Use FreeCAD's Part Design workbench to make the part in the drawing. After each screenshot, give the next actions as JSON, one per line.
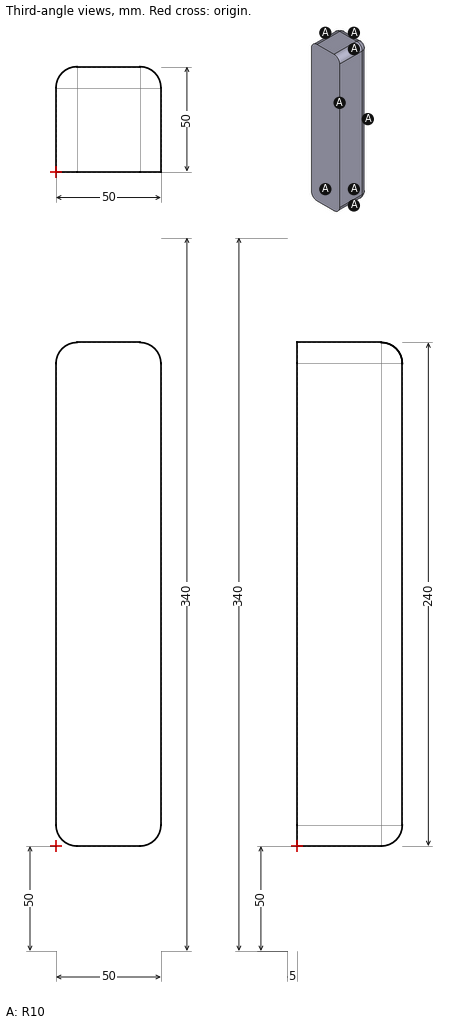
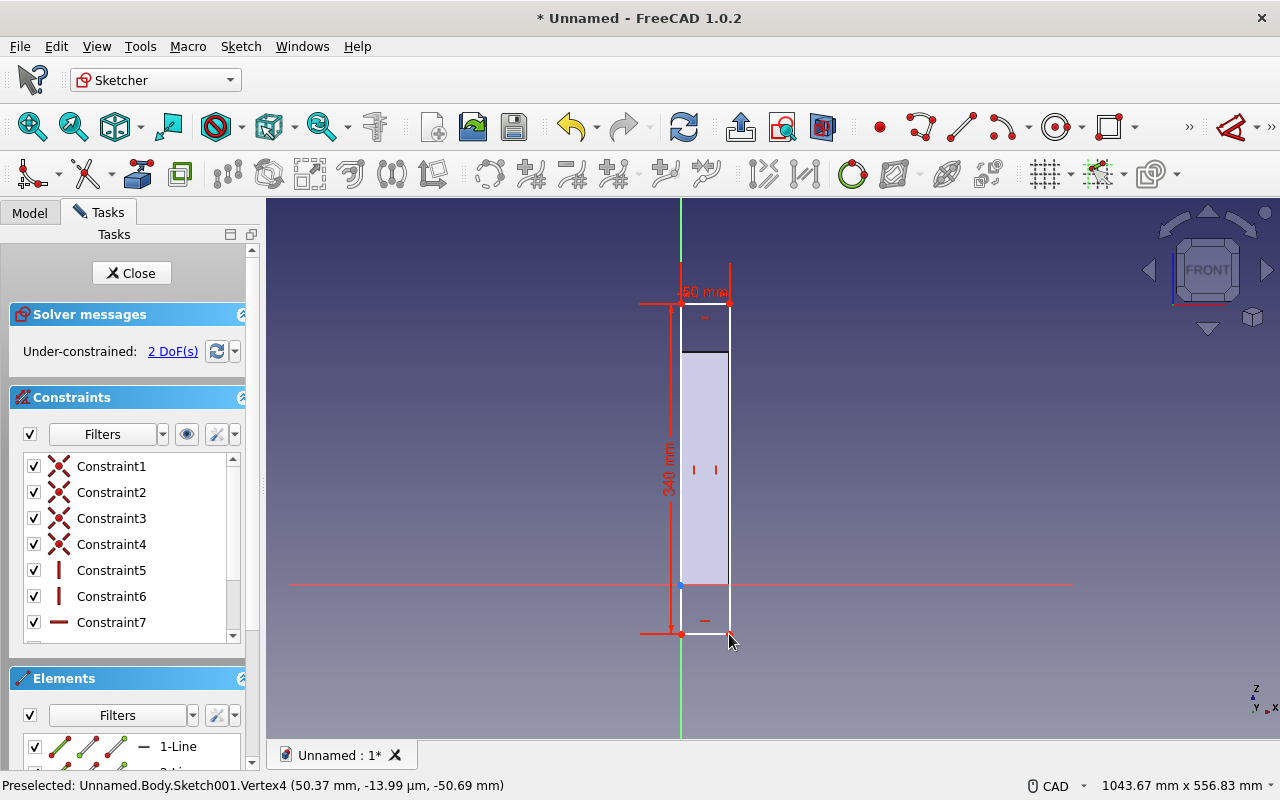
{"action": "left_click", "coordinate": [681, 304]}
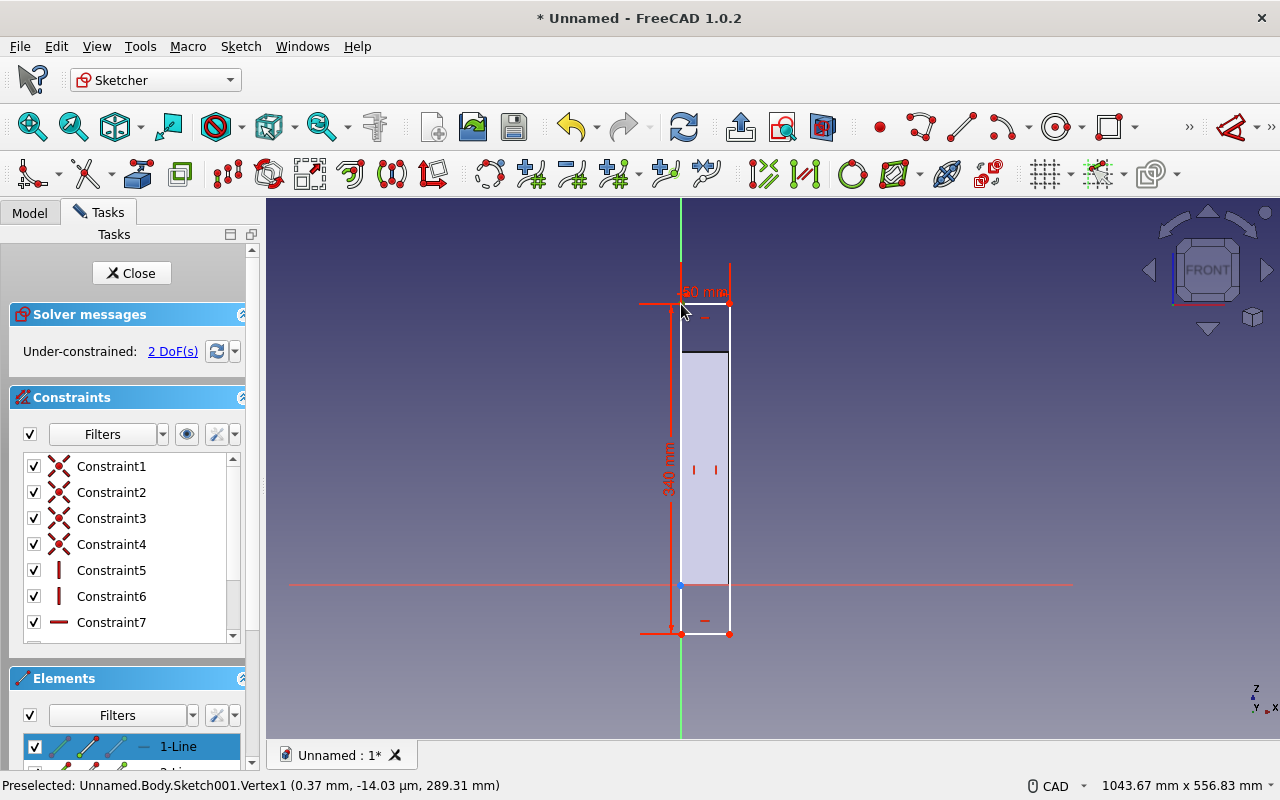
{"action": "left_click", "coordinate": [681, 676]}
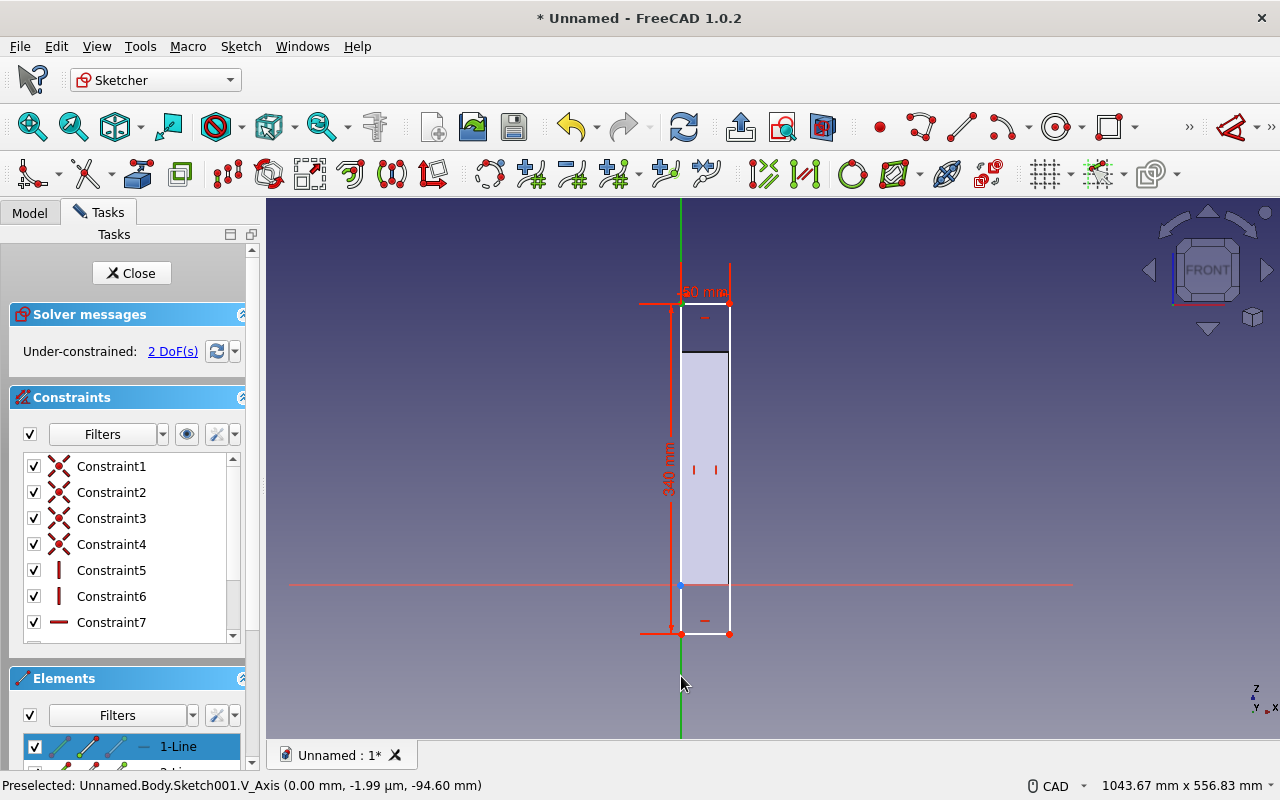
{"action": "key", "text": "c"}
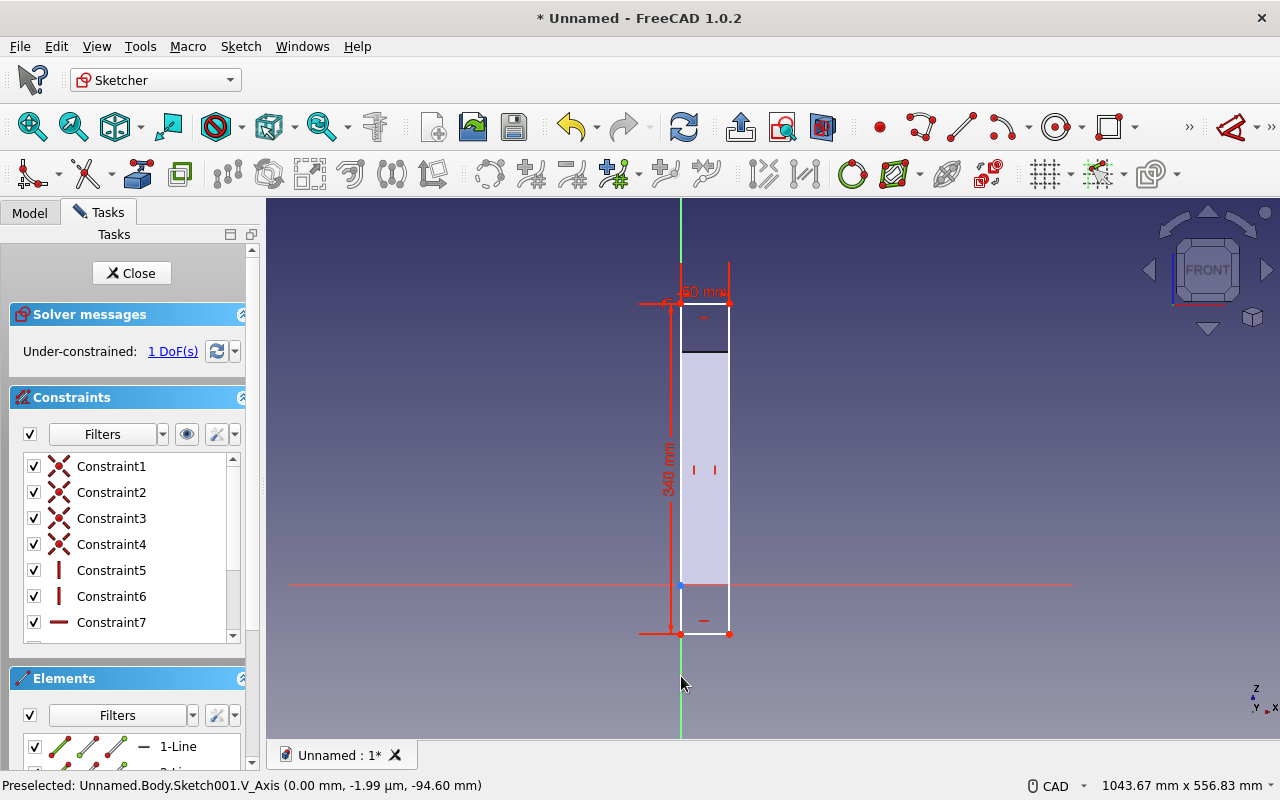
{"action": "left_click", "coordinate": [1230, 128]}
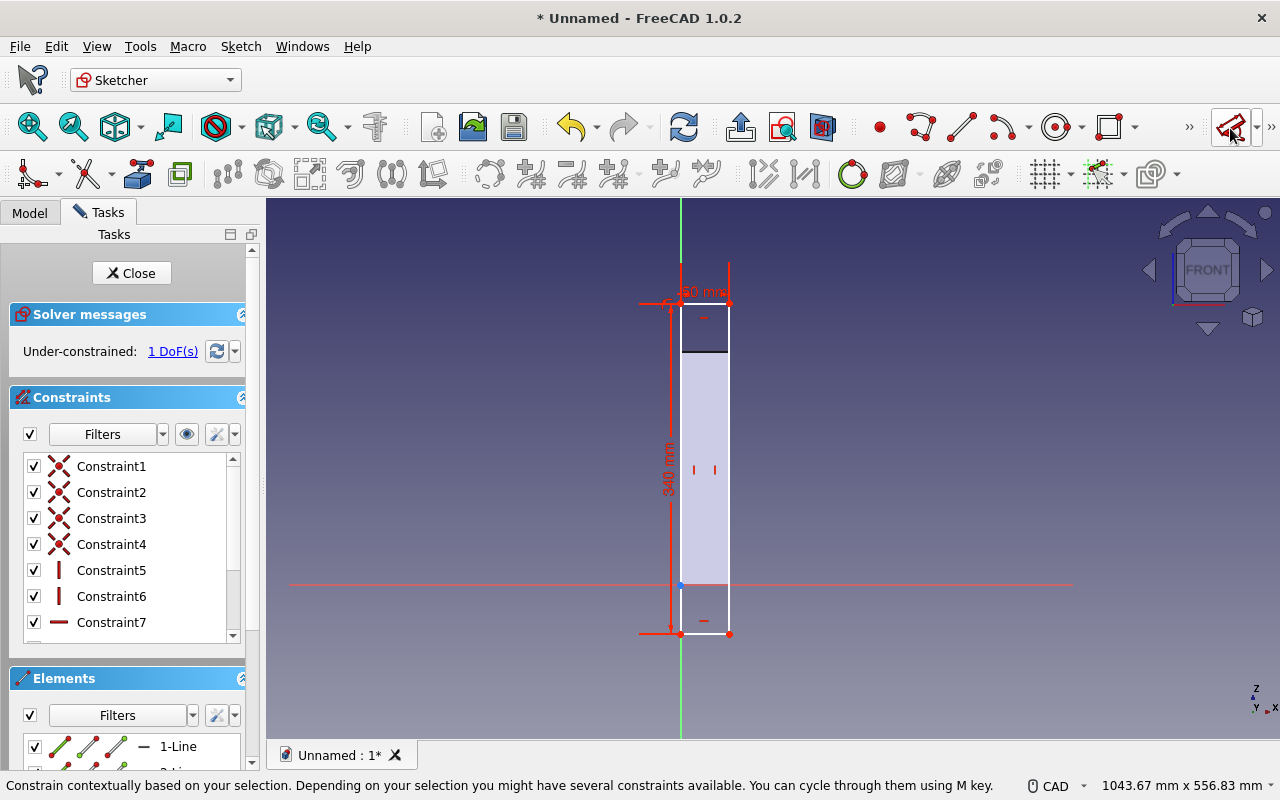
{"action": "left_click", "coordinate": [681, 634]}
{"action": "left_click", "coordinate": [647, 610]}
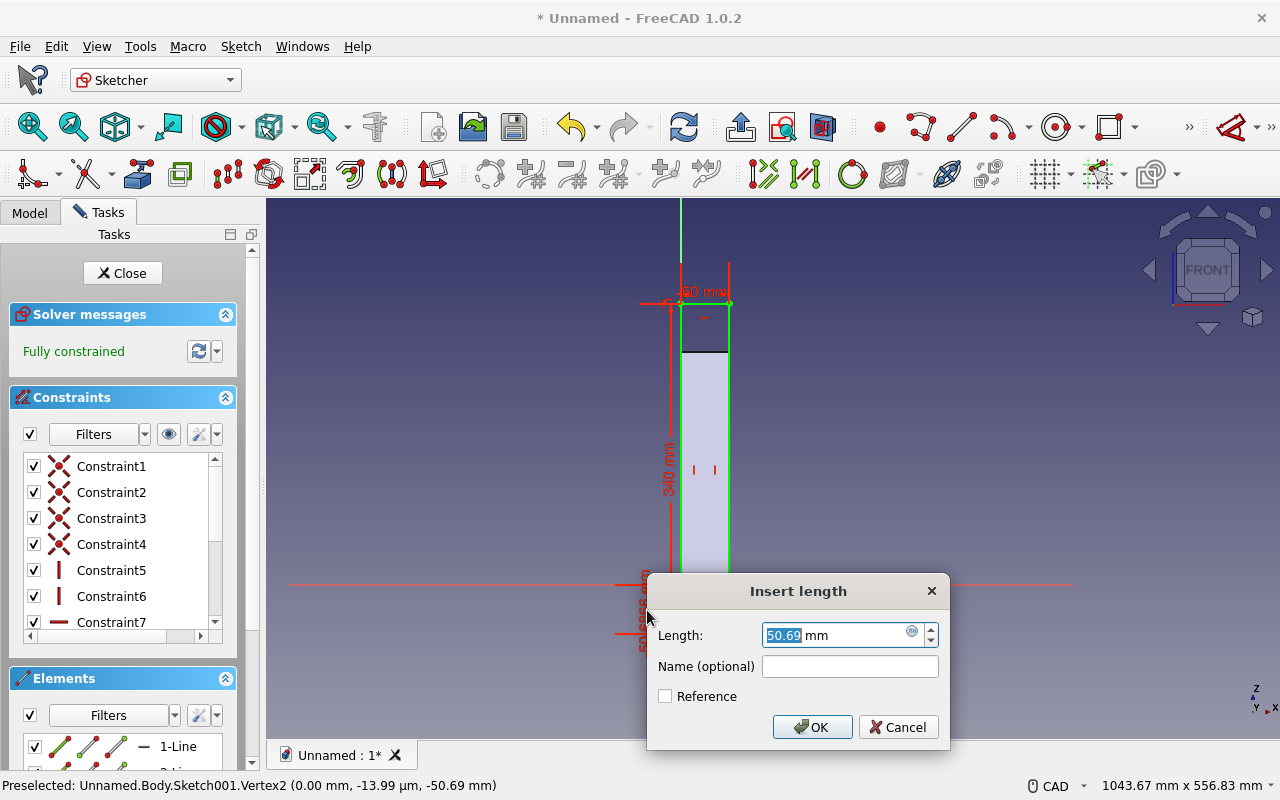
{"action": "type", "text": "50"}
{"action": "key", "text": "Return"}
{"action": "key", "text": "Escape"}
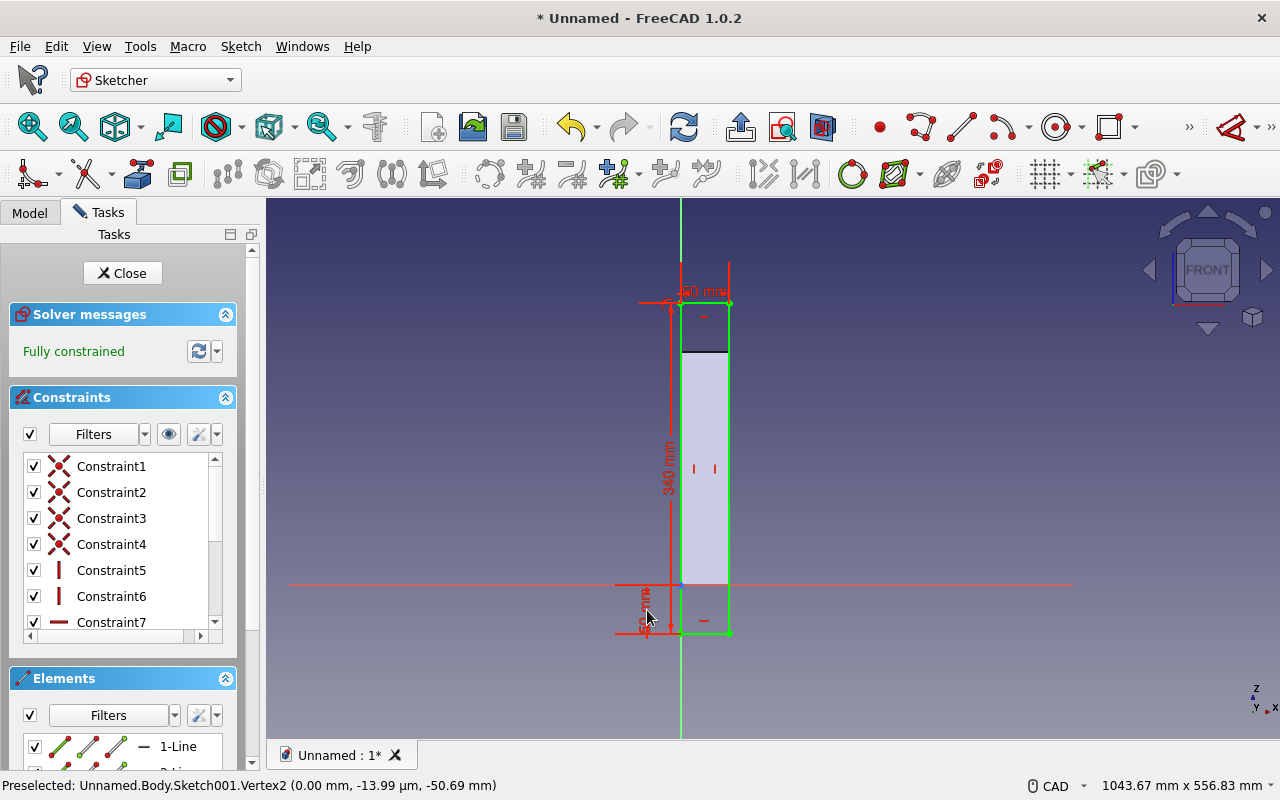
{"action": "left_click", "coordinate": [123, 273]}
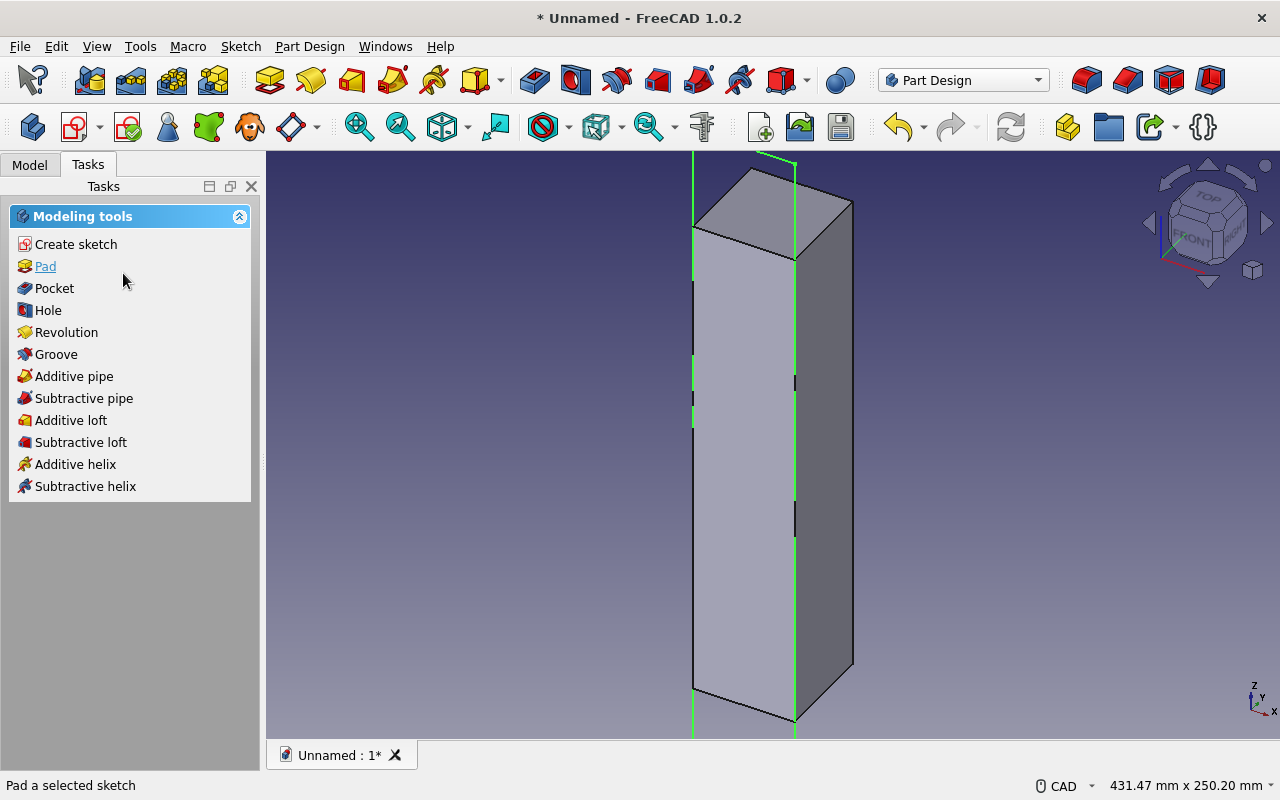
{"action": "left_click", "coordinate": [270, 80]}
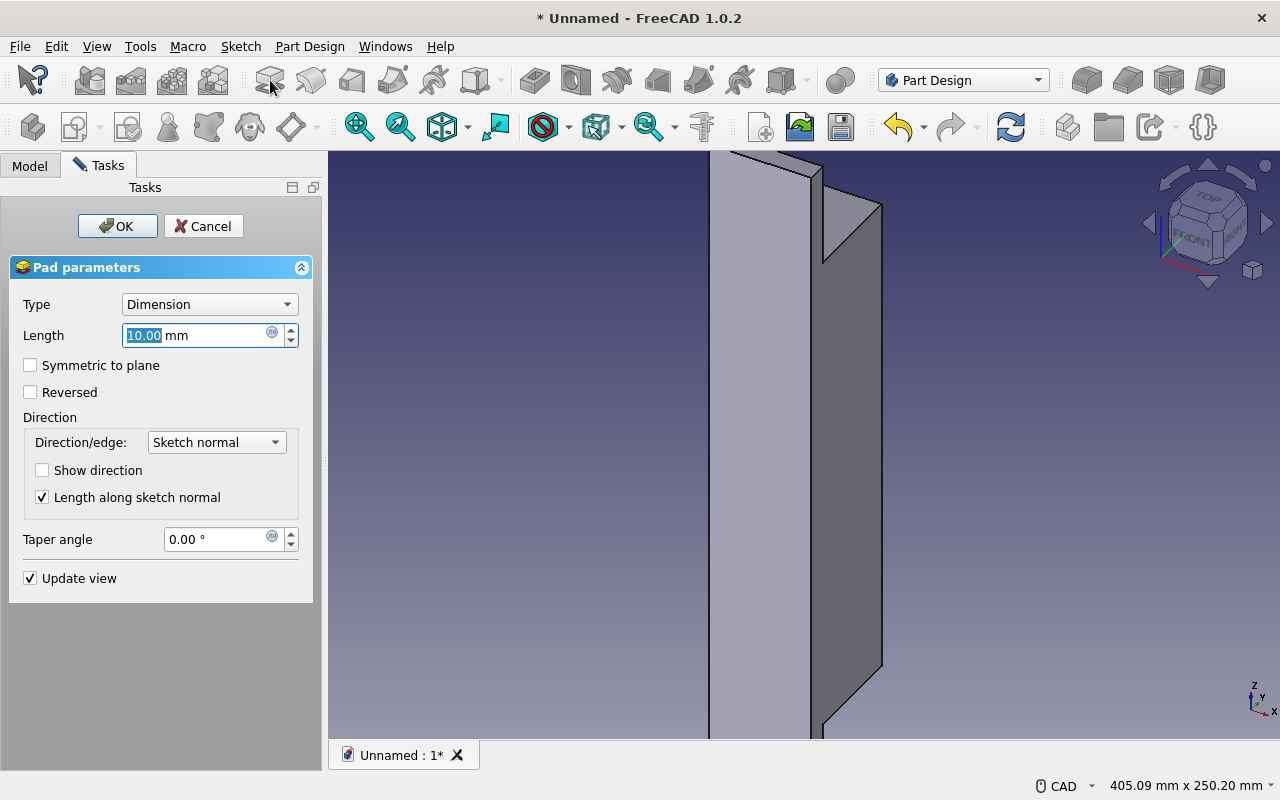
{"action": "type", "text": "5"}
{"action": "key", "text": "Tab"}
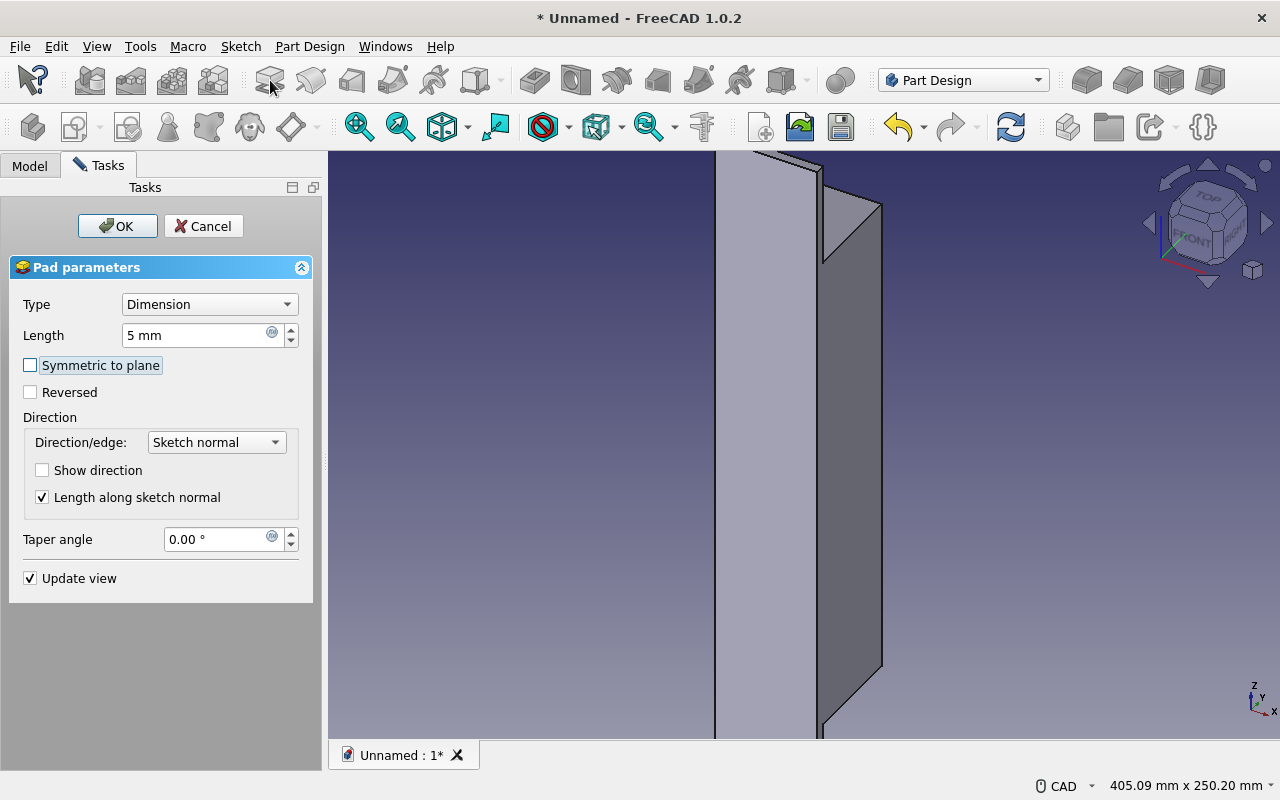
{"action": "left_click", "coordinate": [118, 226]}